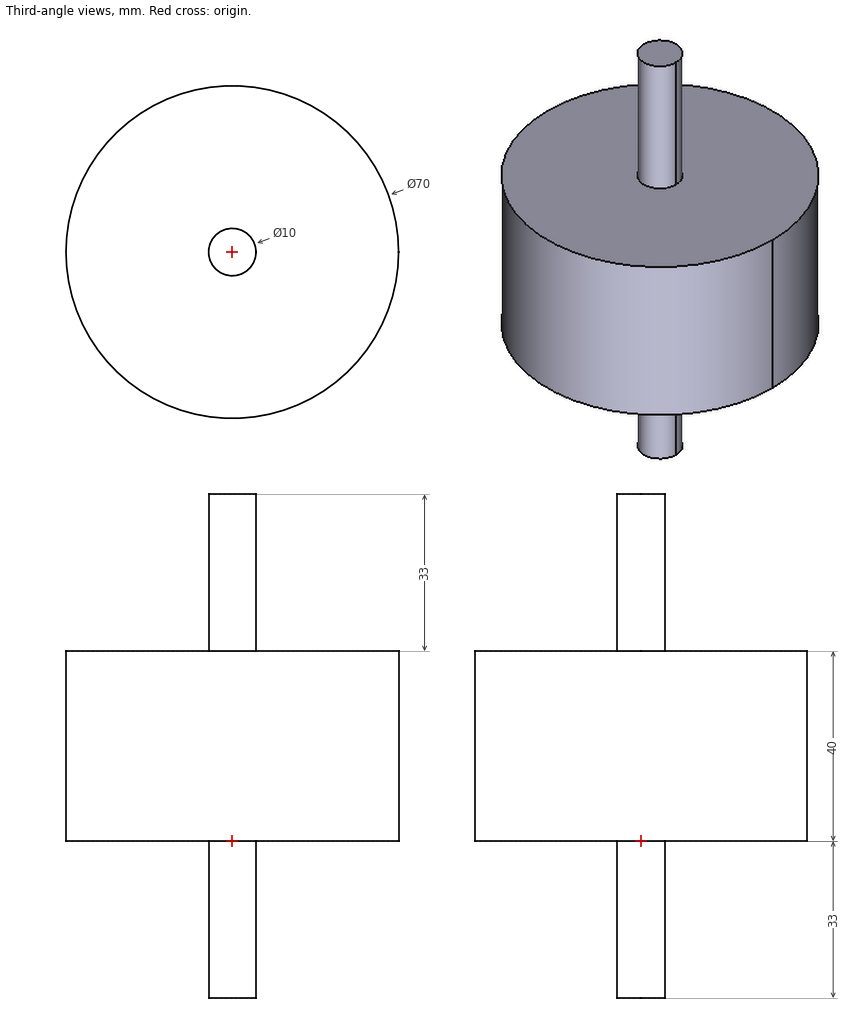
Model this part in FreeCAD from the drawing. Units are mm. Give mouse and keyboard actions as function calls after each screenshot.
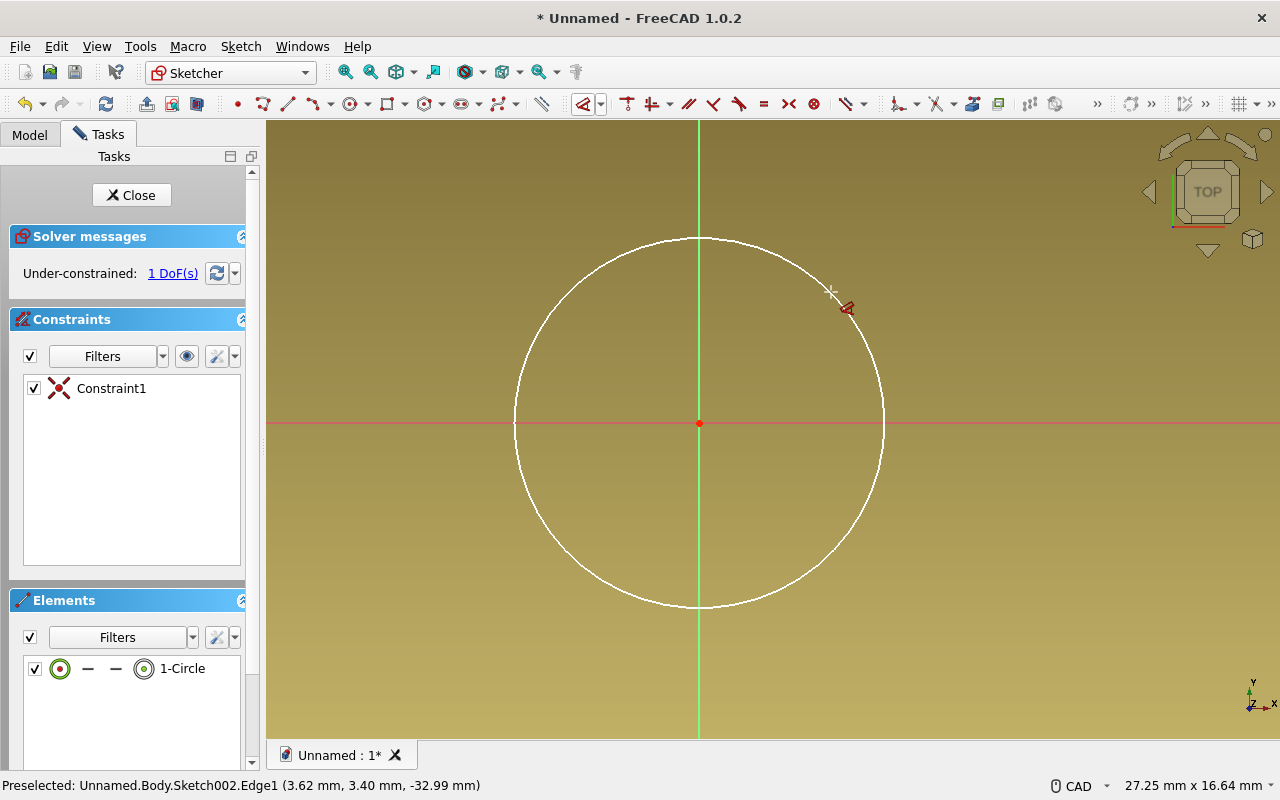
click(830, 292)
click(853, 269)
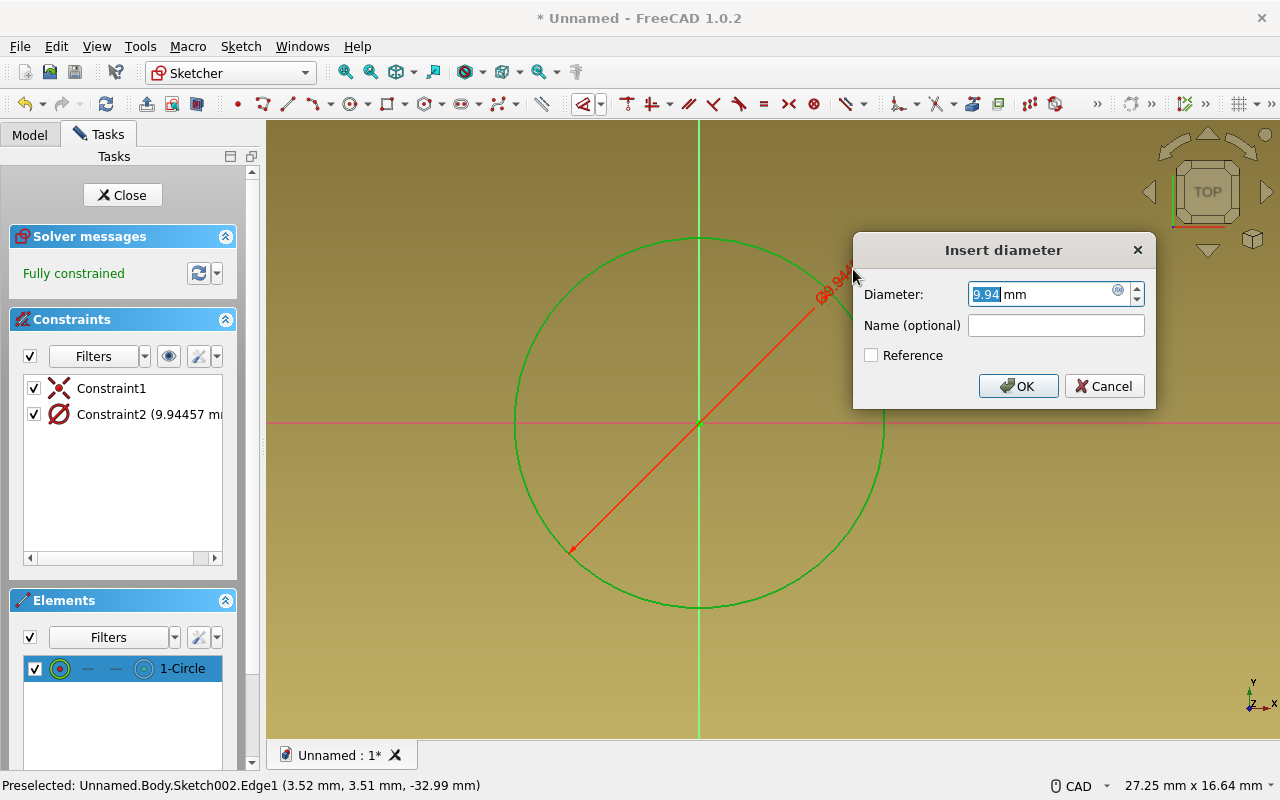
text(10)
key(Return)
key(Escape)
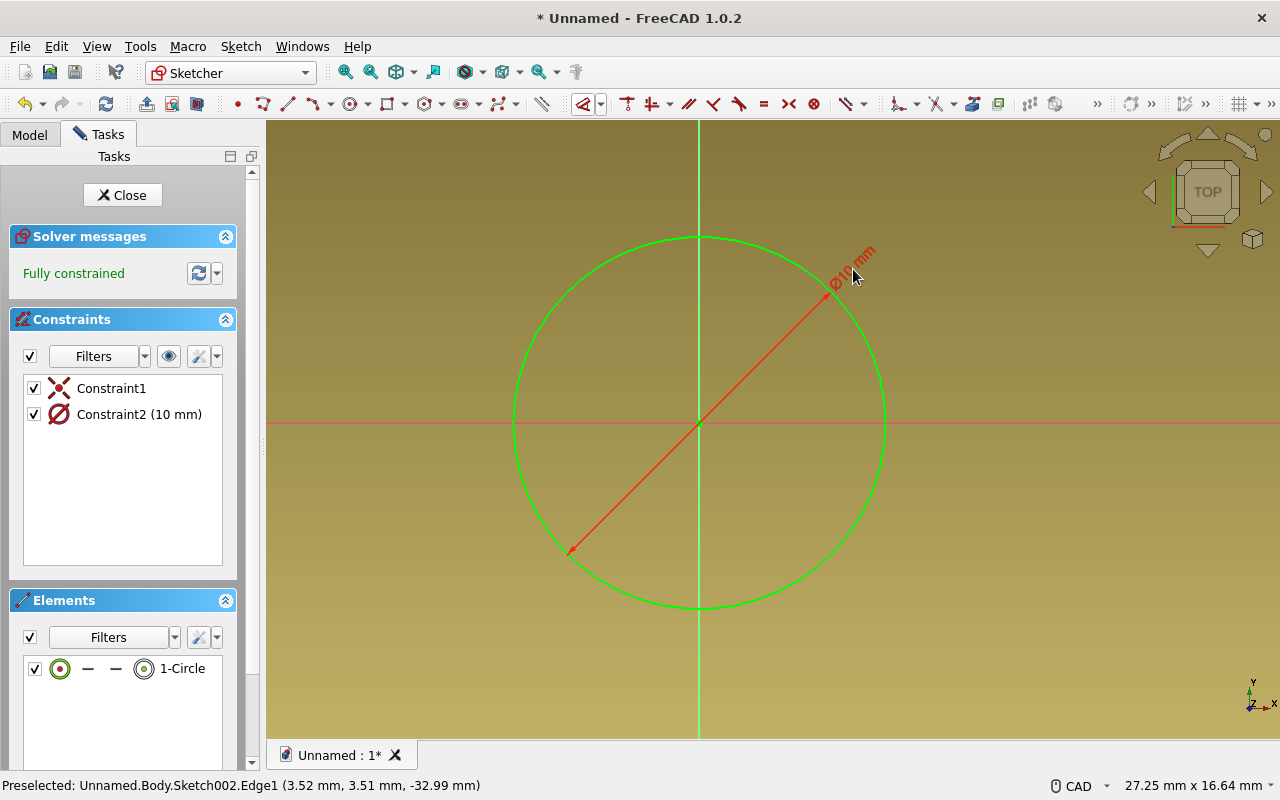
click(123, 195)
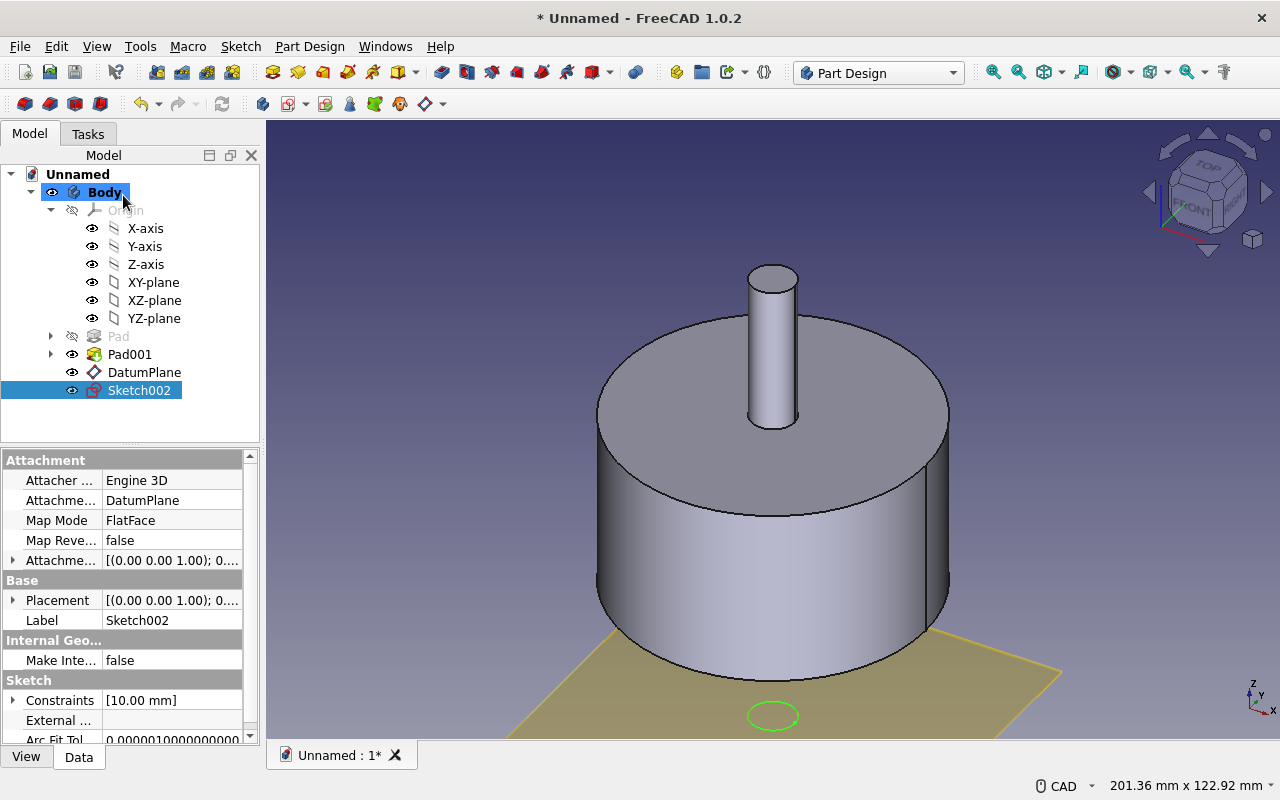
click(273, 72)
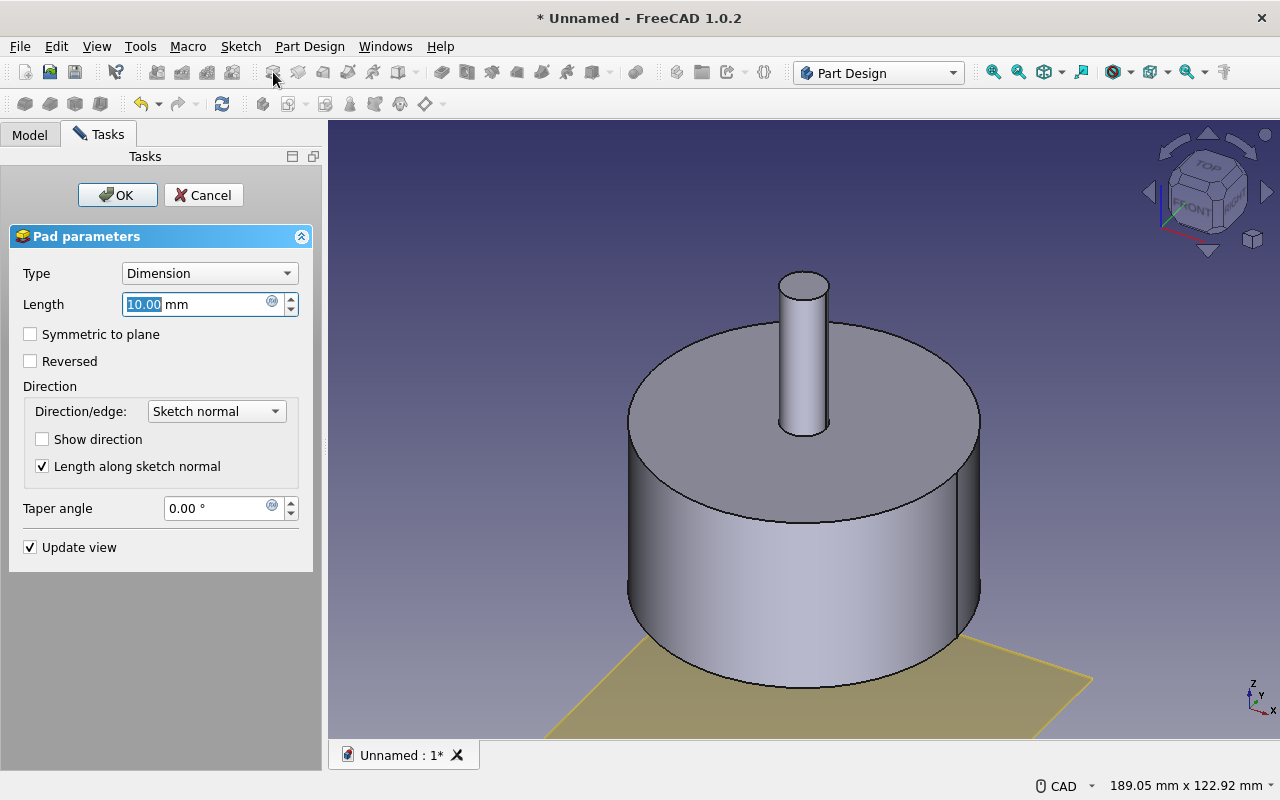
text(33)
key(Tab)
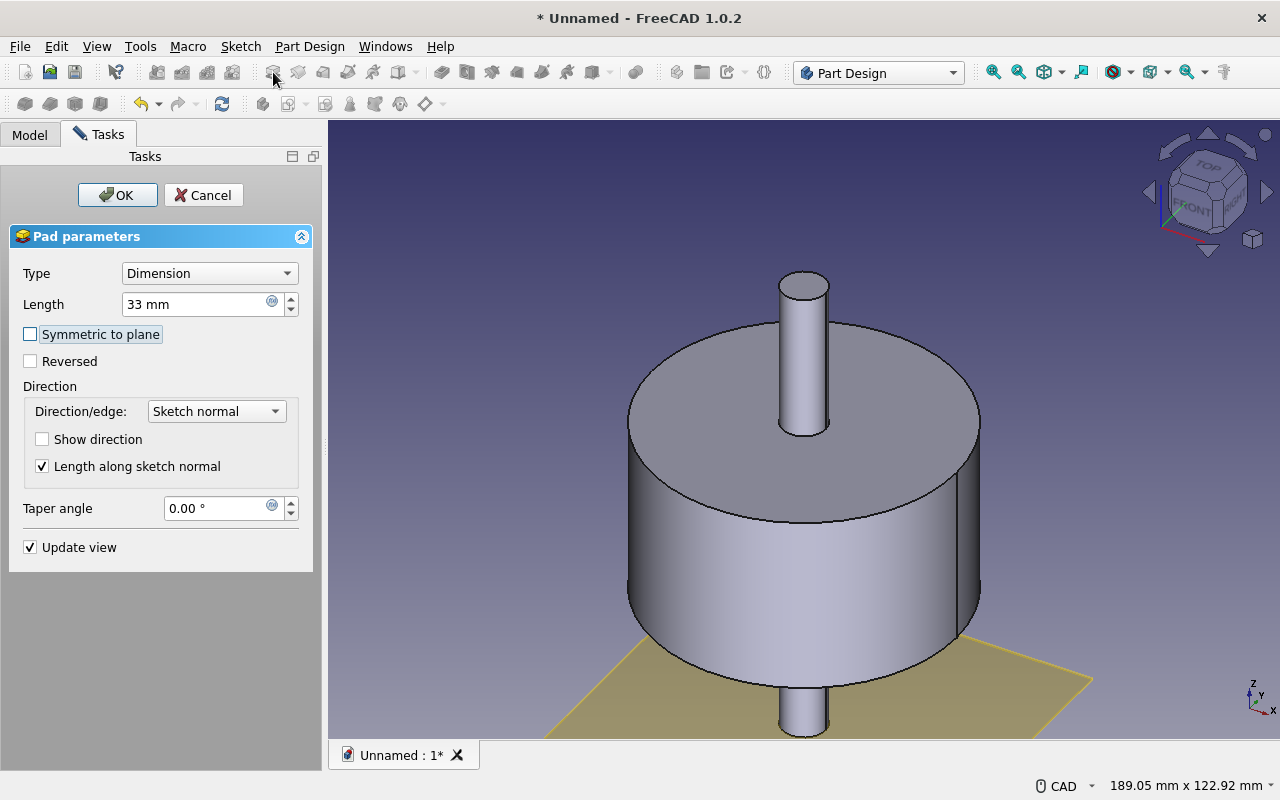
click(118, 195)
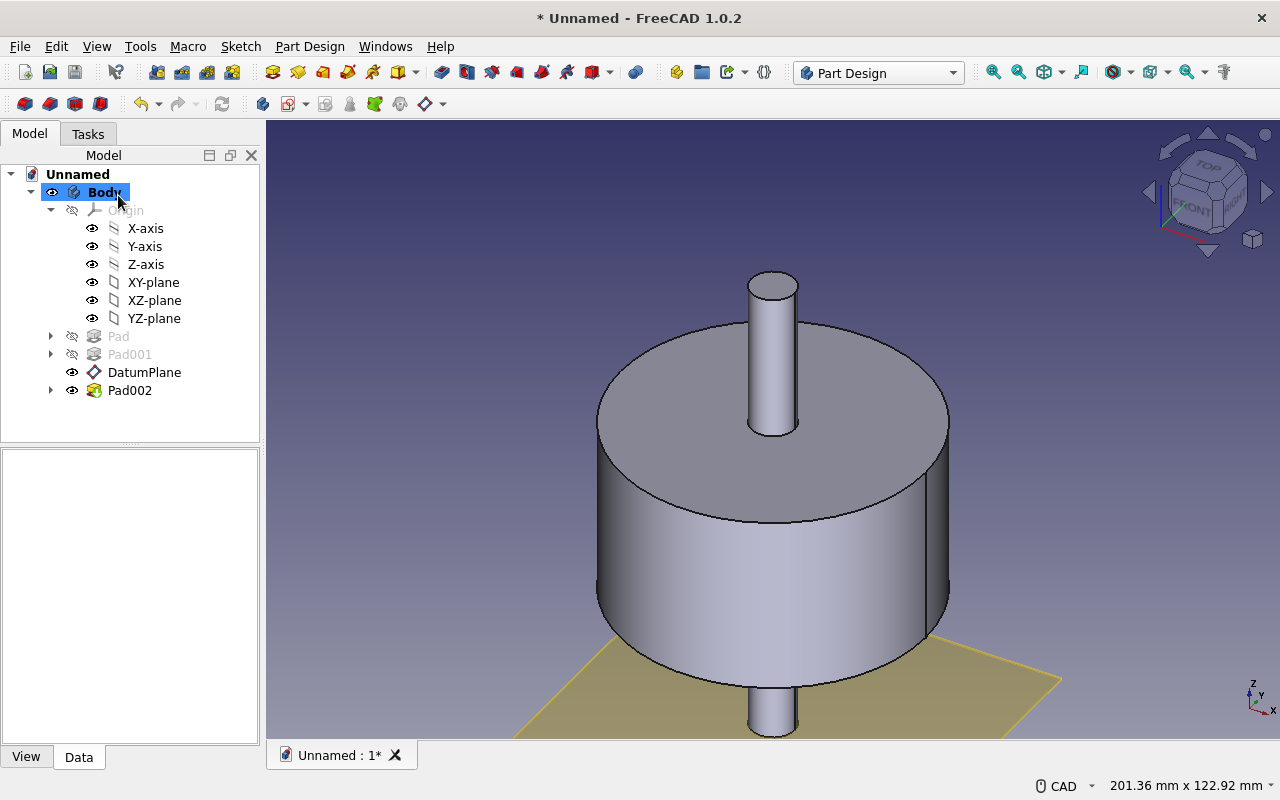
click(117, 372)
key(space)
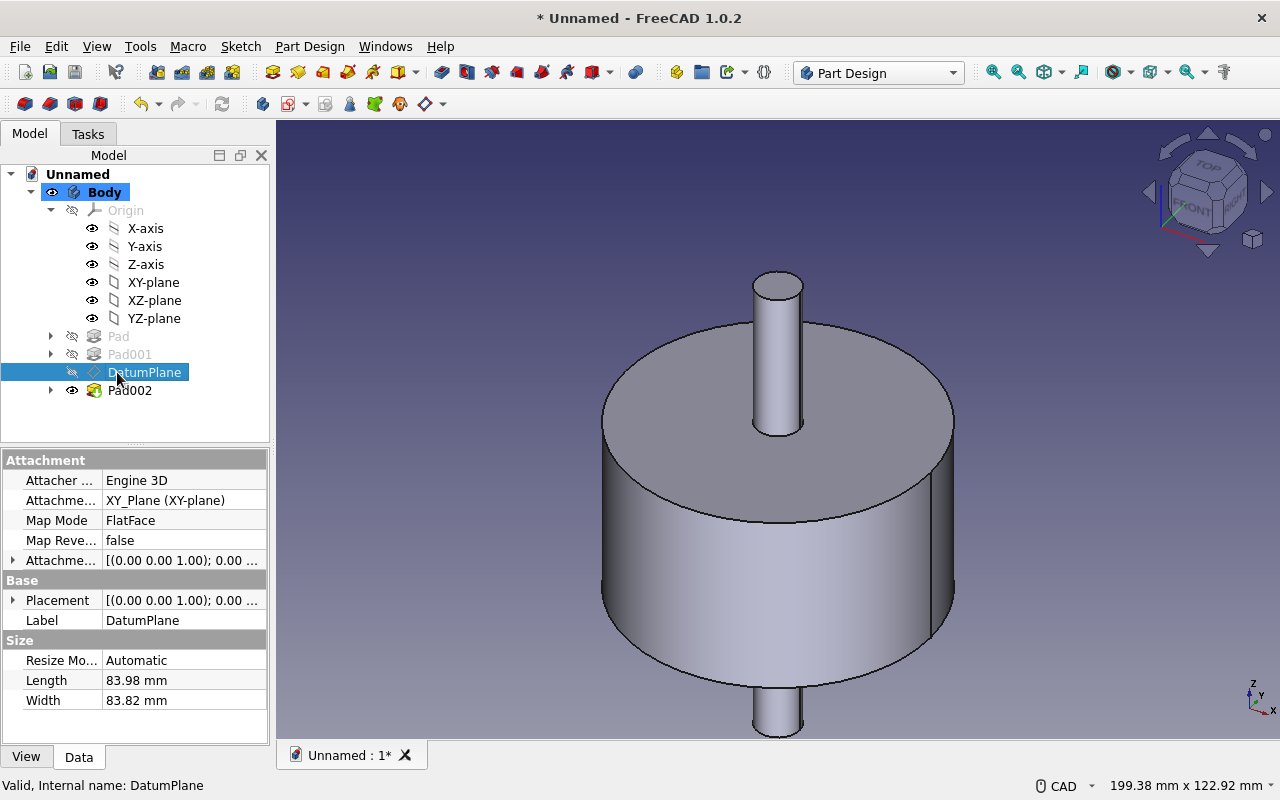
key(0)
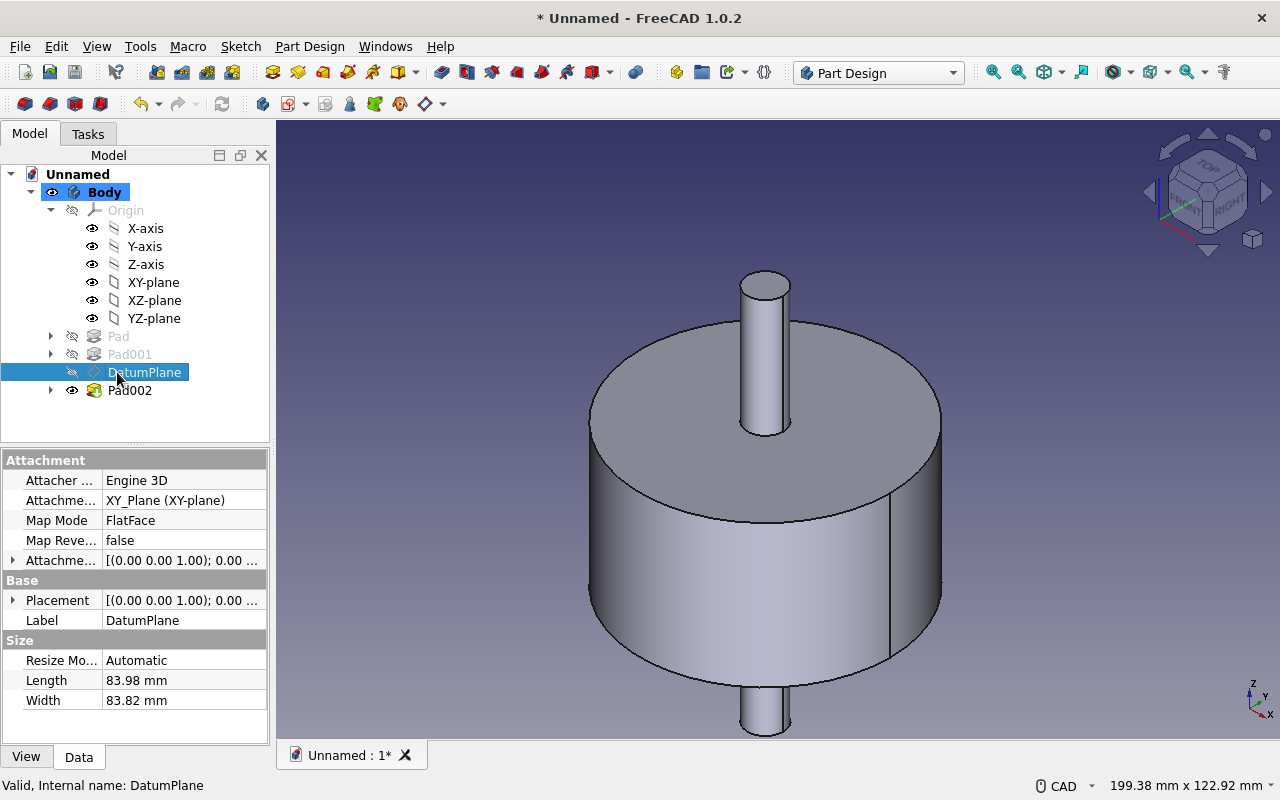
key(v)
key(f)